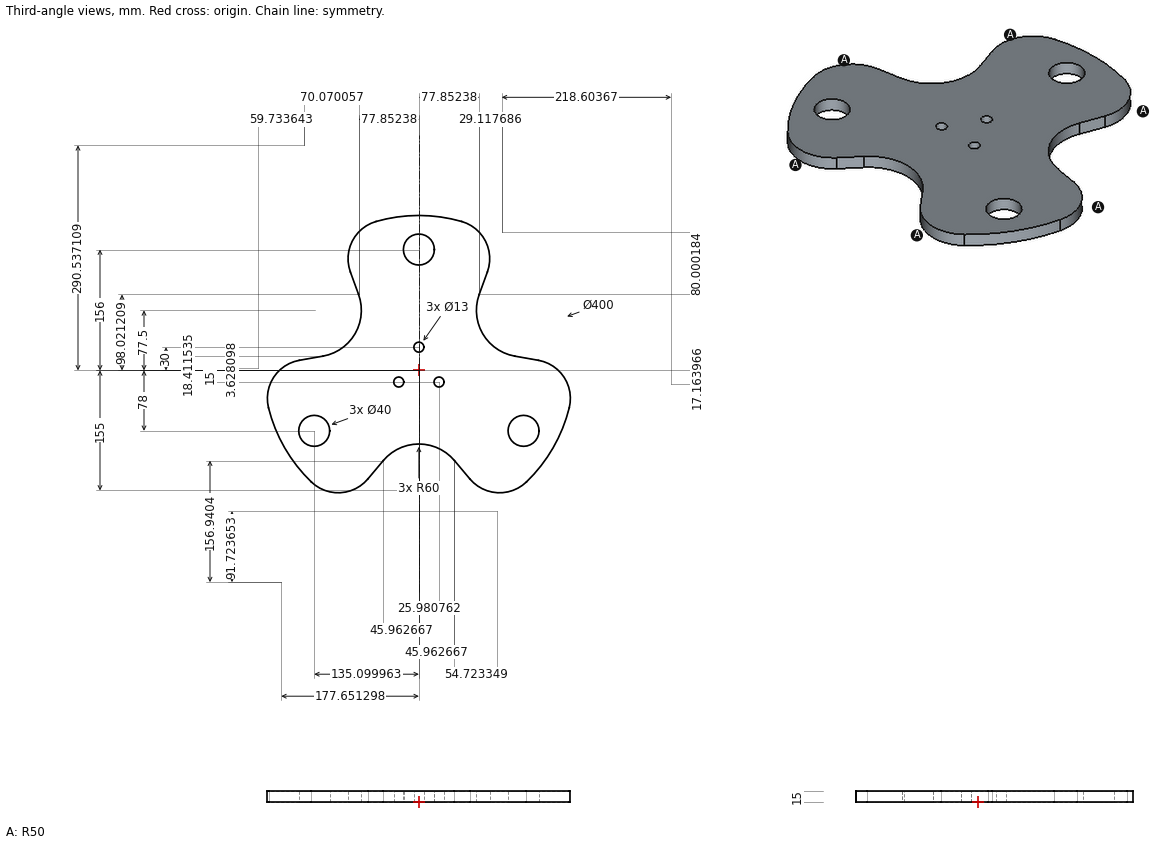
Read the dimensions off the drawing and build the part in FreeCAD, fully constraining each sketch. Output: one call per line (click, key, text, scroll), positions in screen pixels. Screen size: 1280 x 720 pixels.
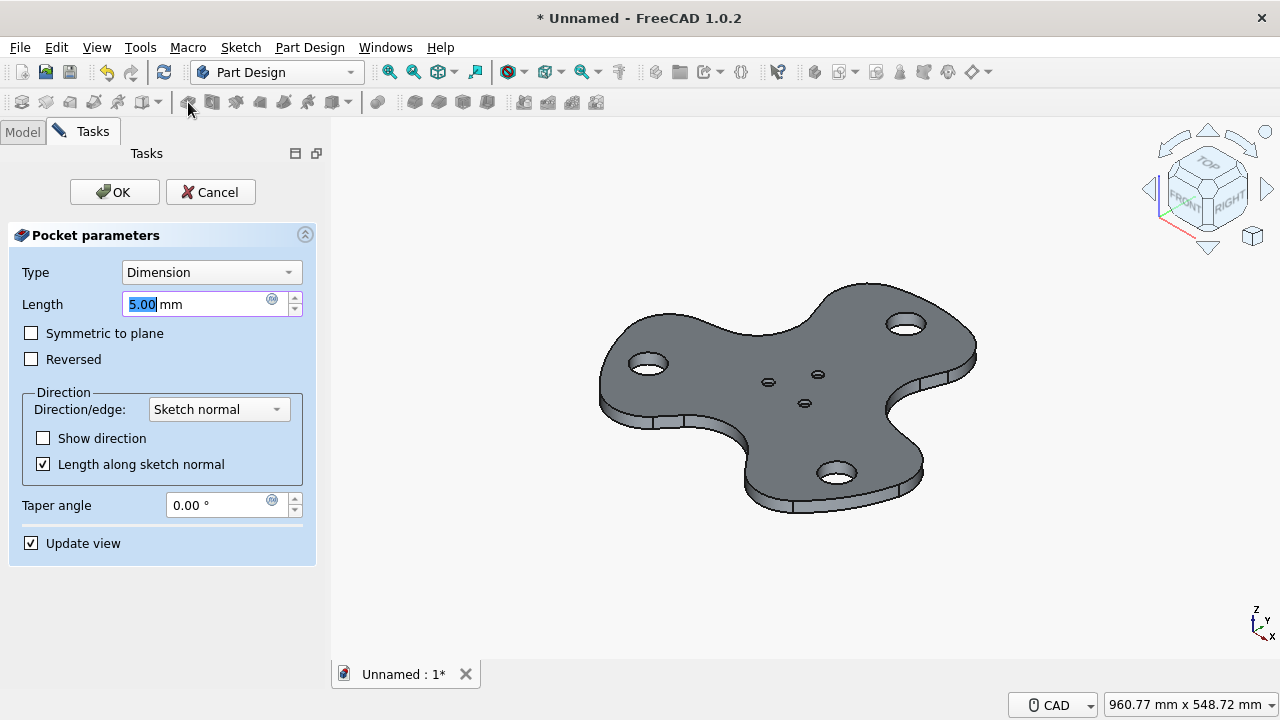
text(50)
key(Tab)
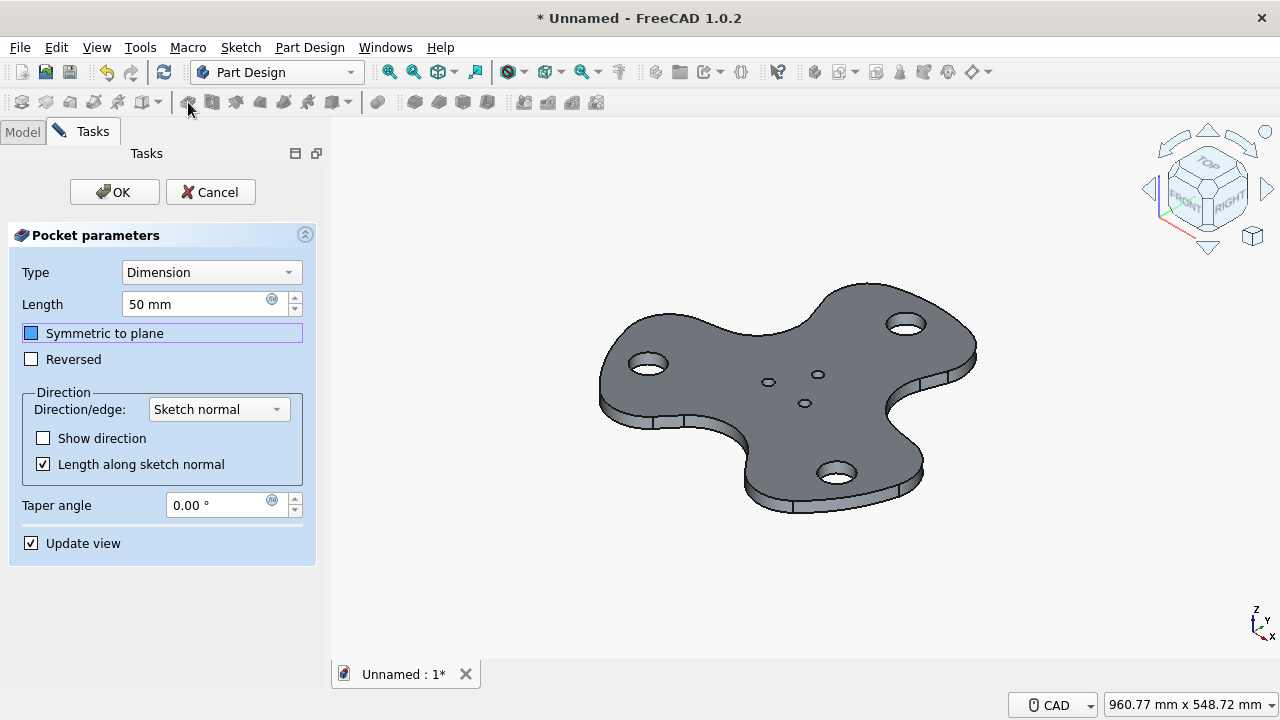
click(115, 192)